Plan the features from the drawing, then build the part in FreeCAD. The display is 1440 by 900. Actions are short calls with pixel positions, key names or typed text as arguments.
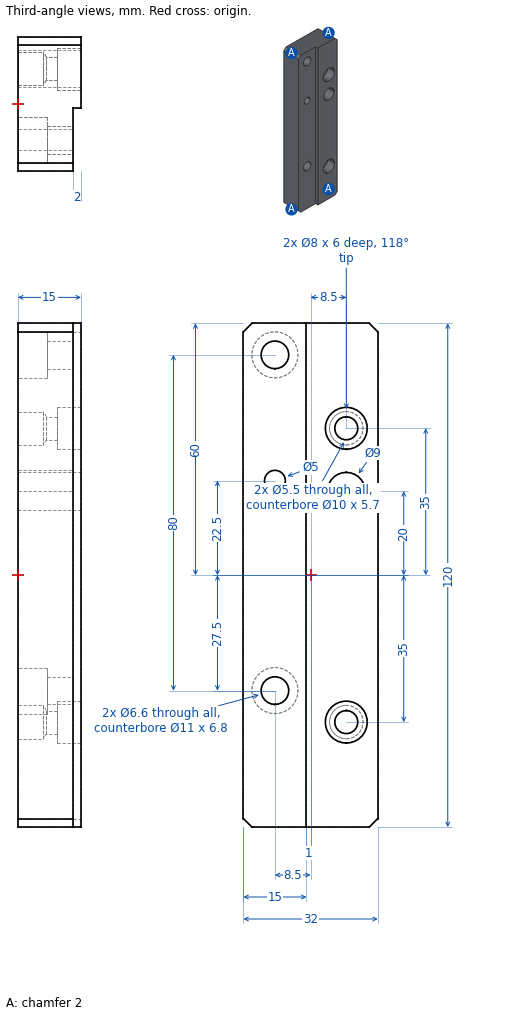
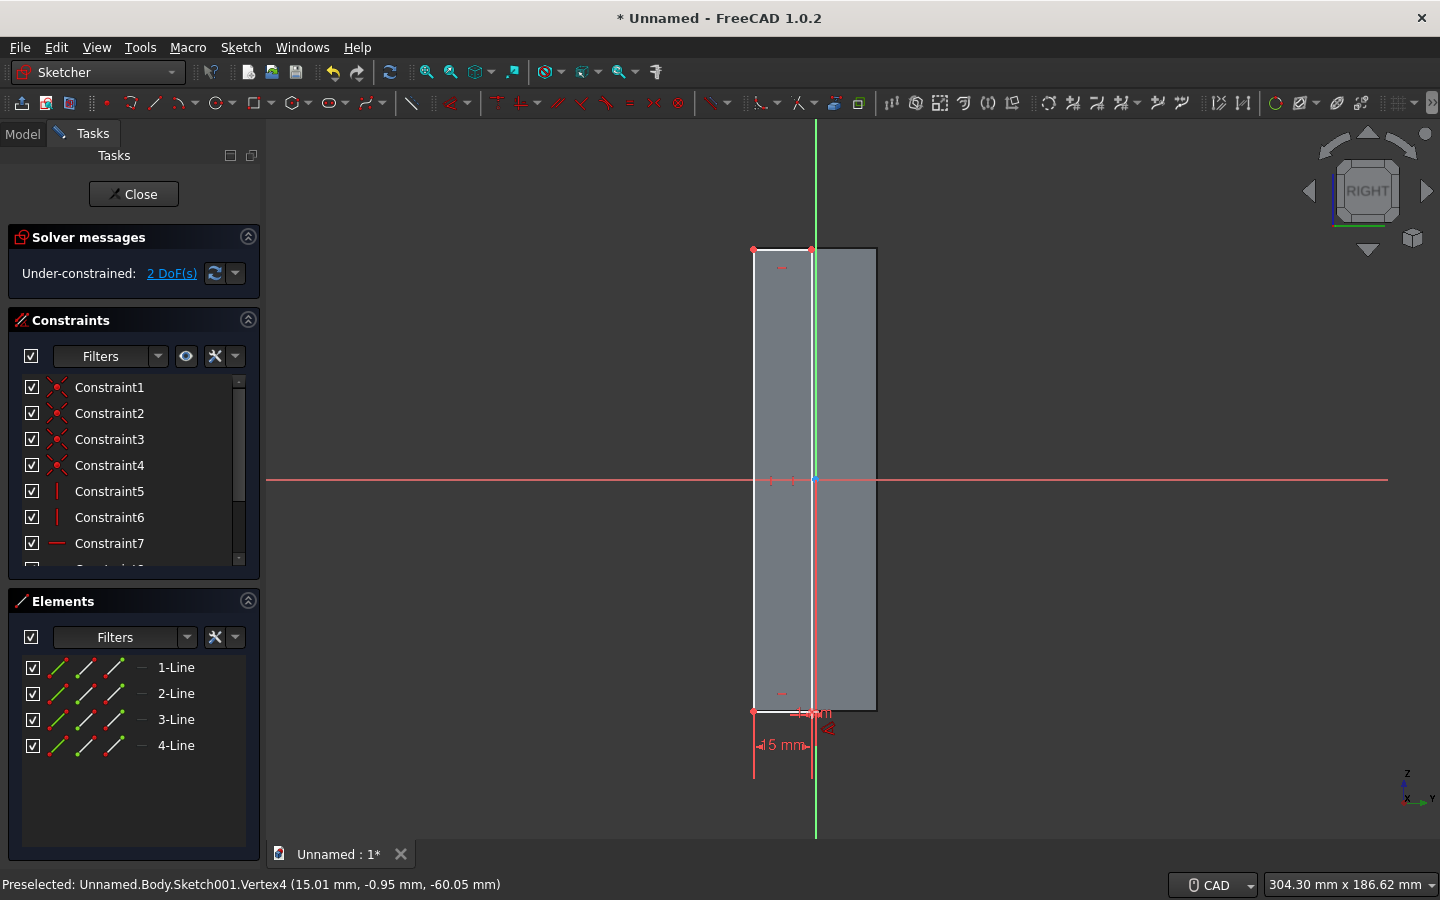
click(754, 388)
click(720, 374)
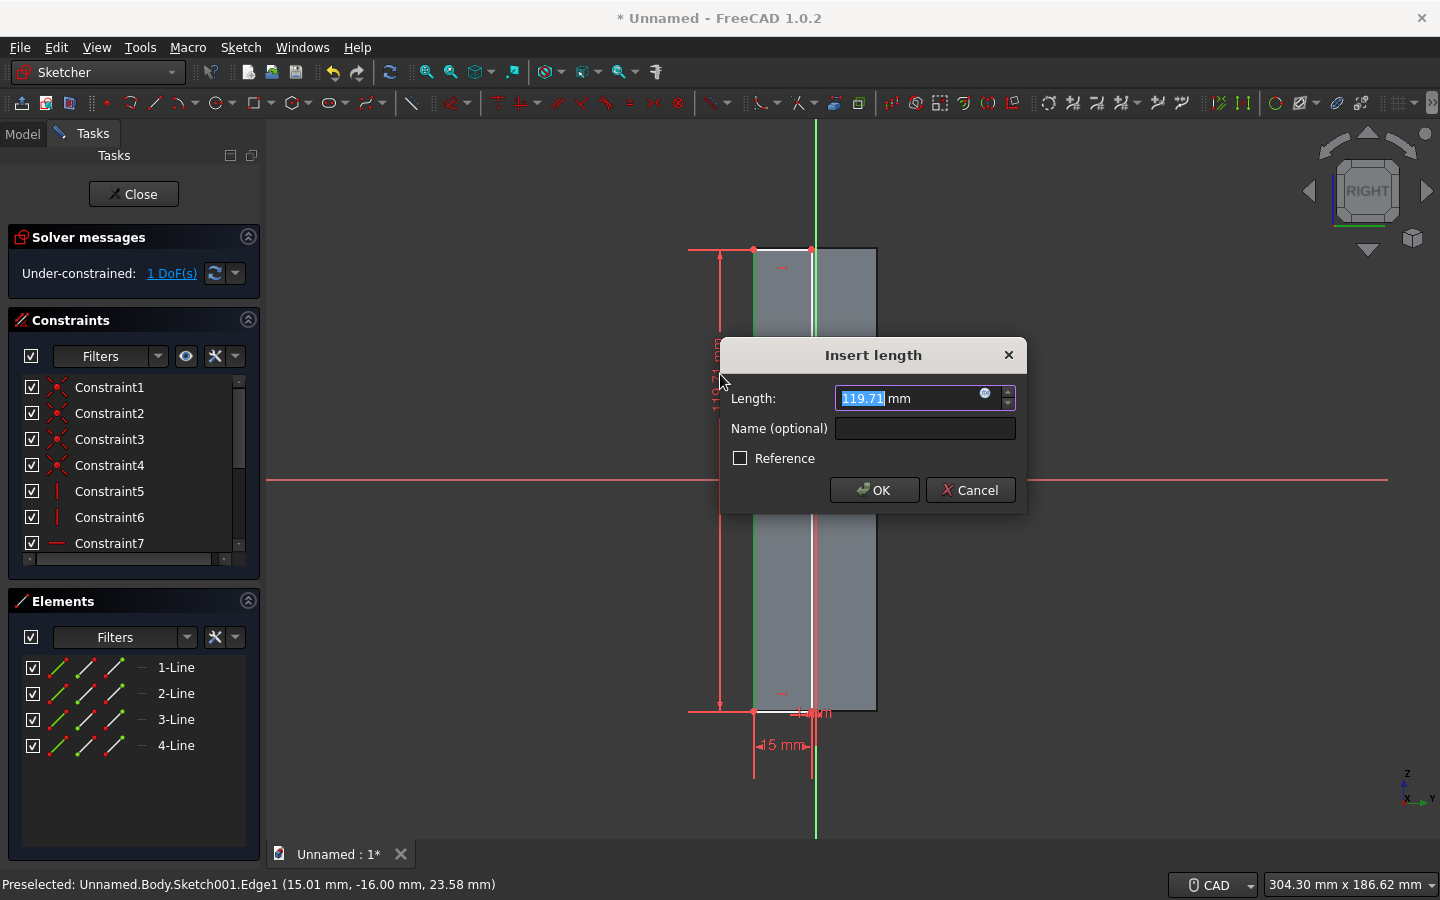
text(120)
key(Return)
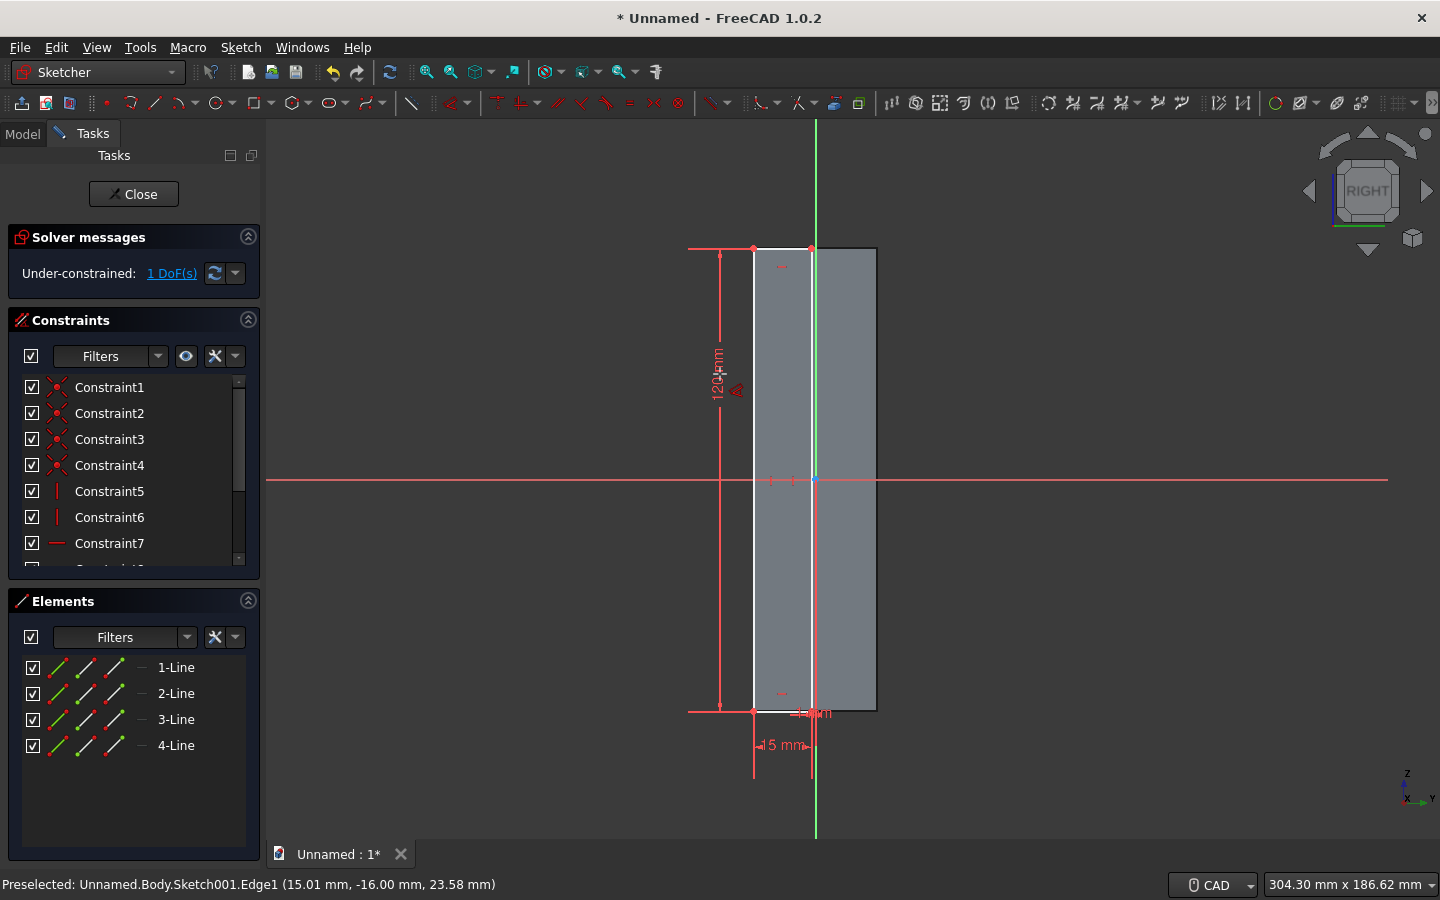
click(754, 249)
click(850, 364)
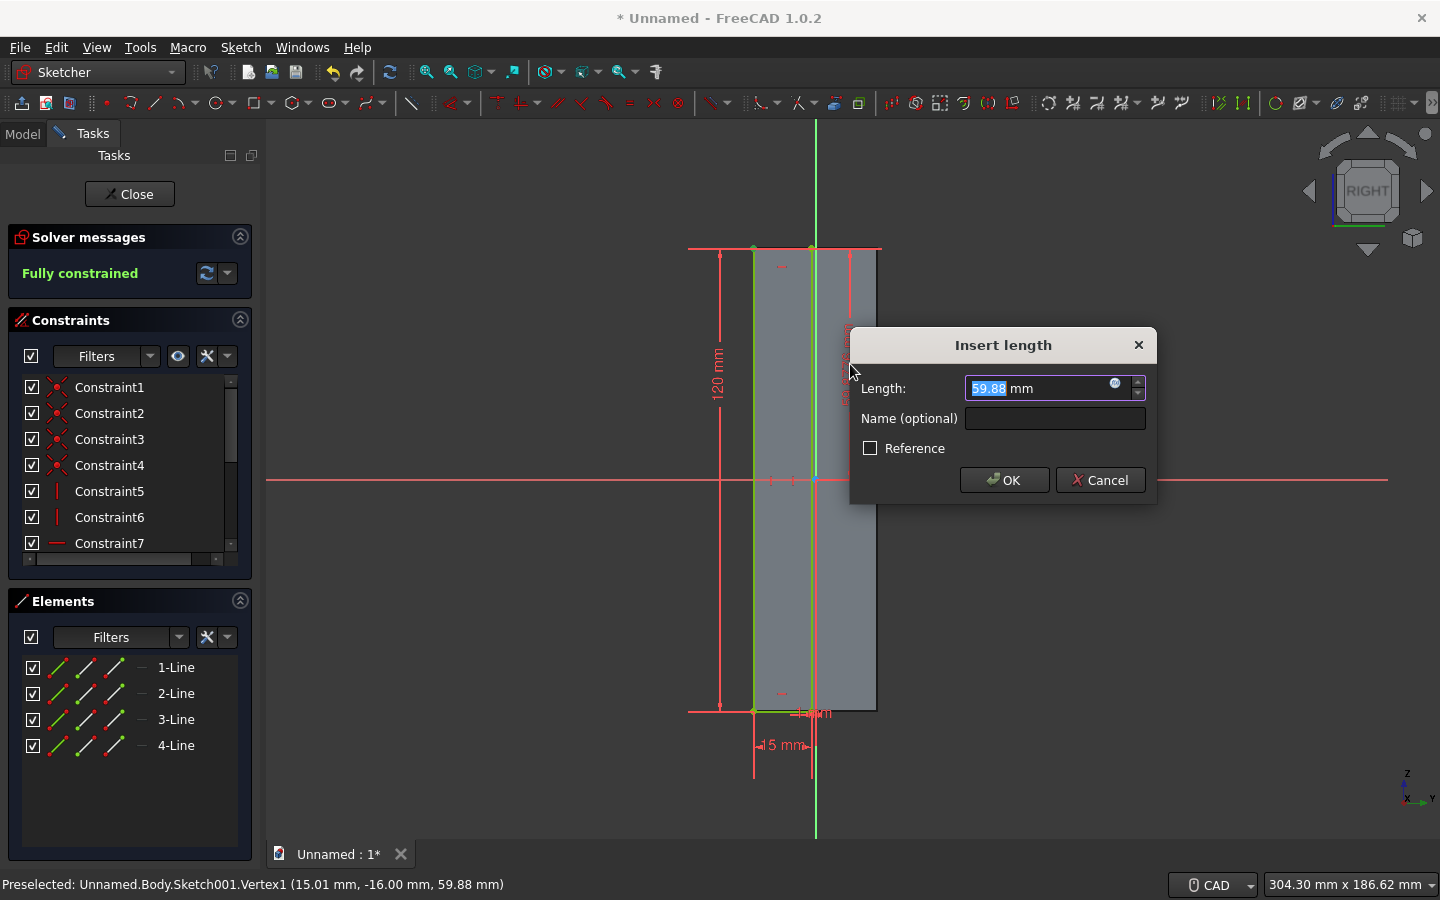
text(60)
key(Return)
key(Escape)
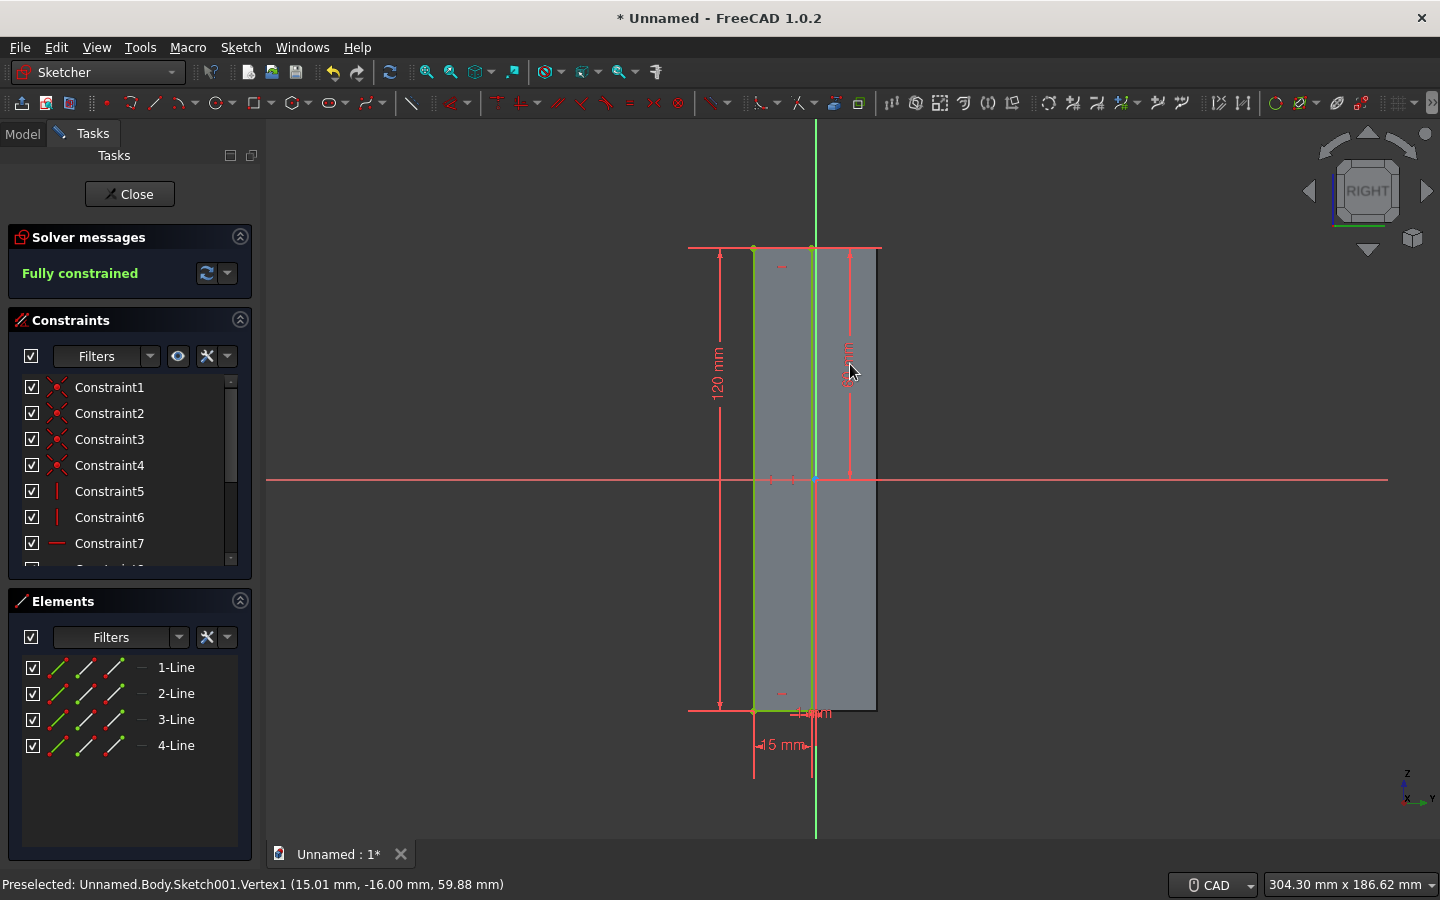
click(130, 194)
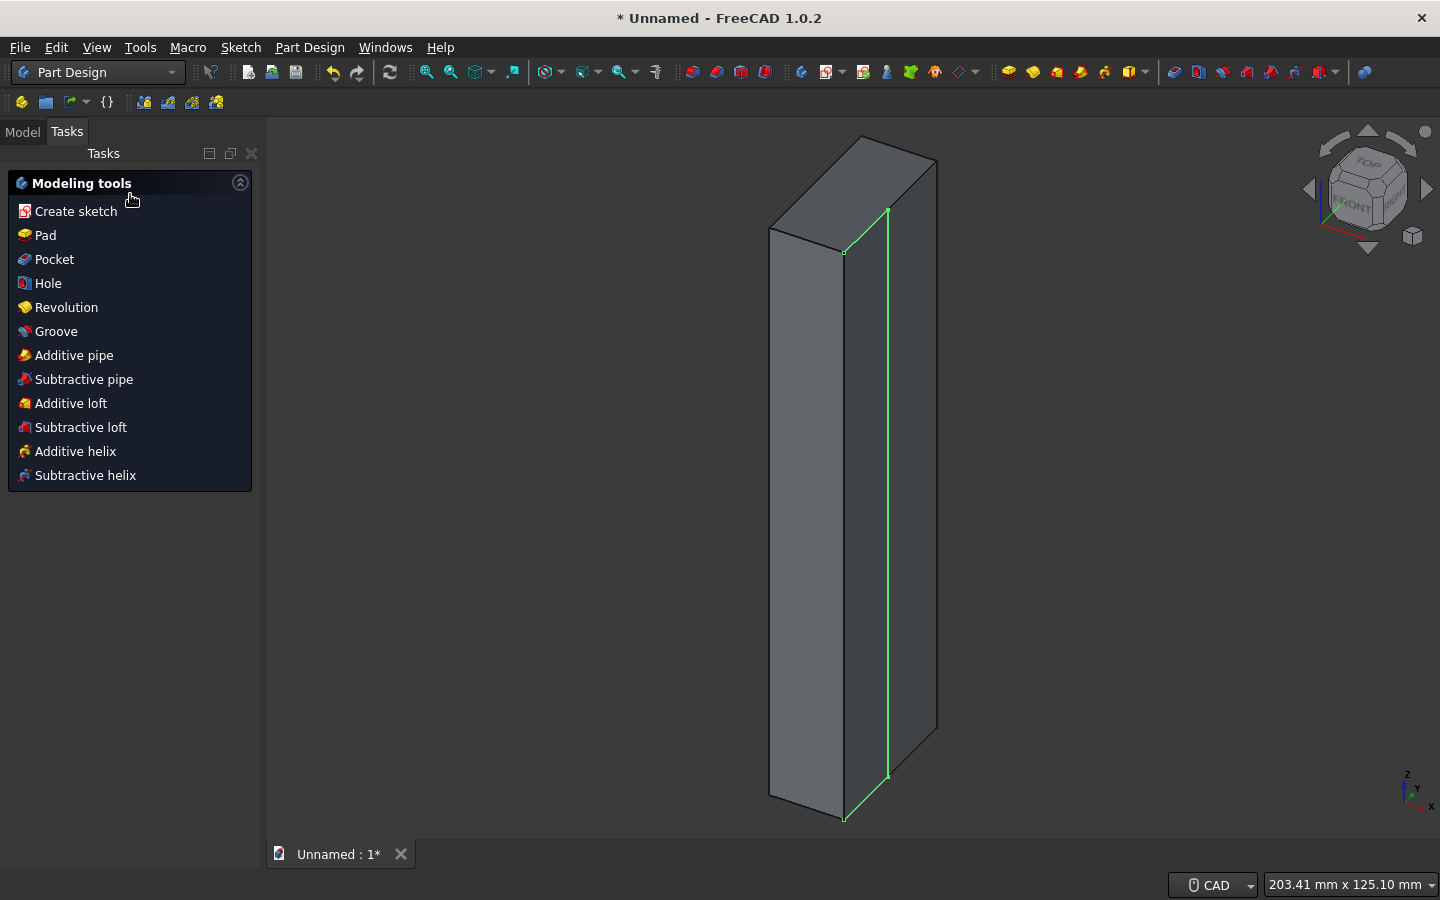
click(1176, 72)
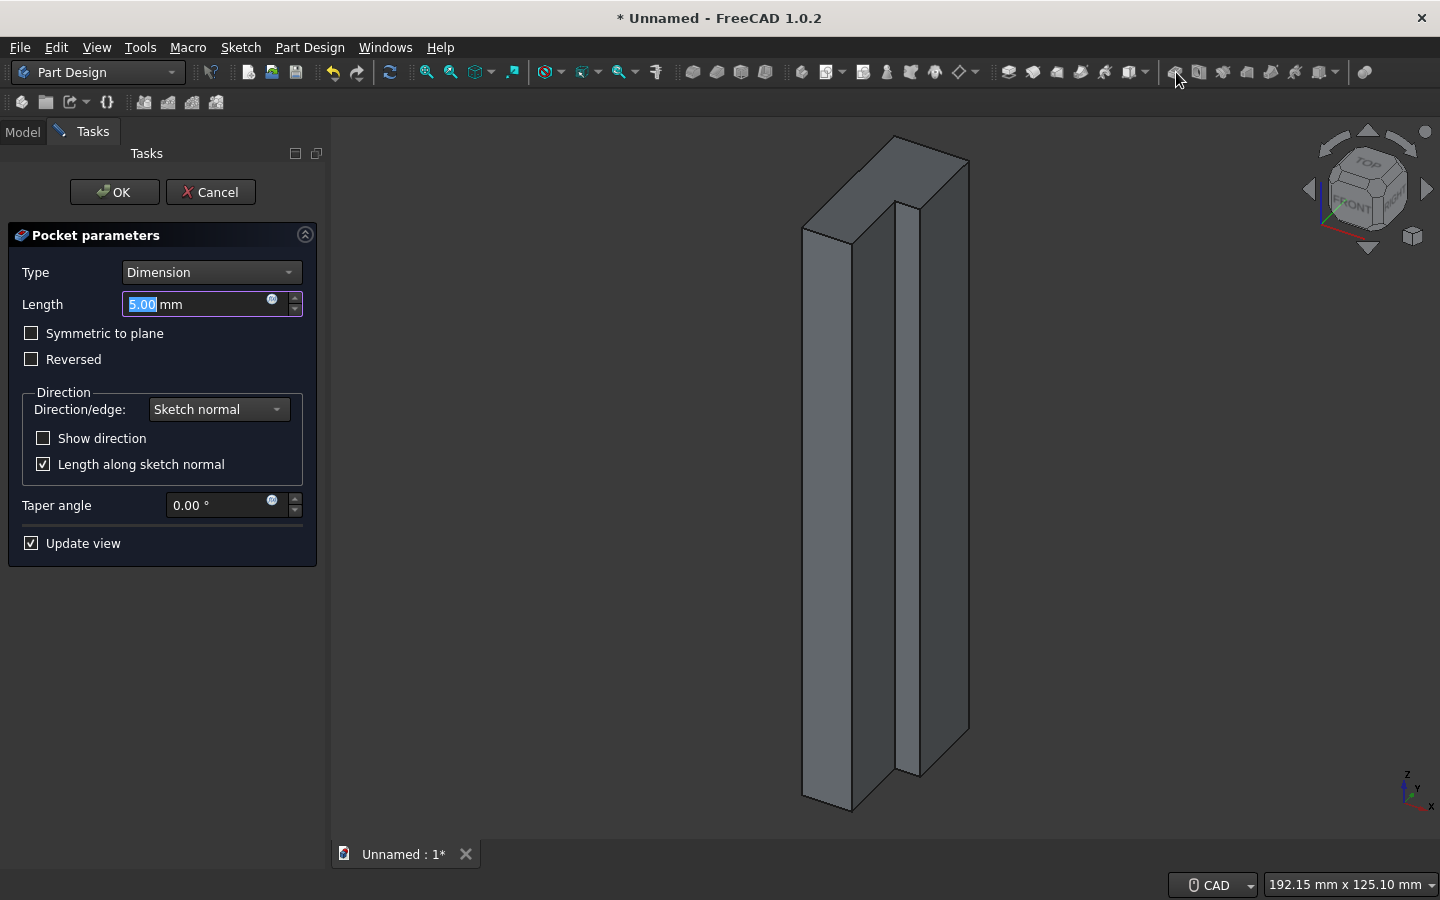
text(2)
key(Tab)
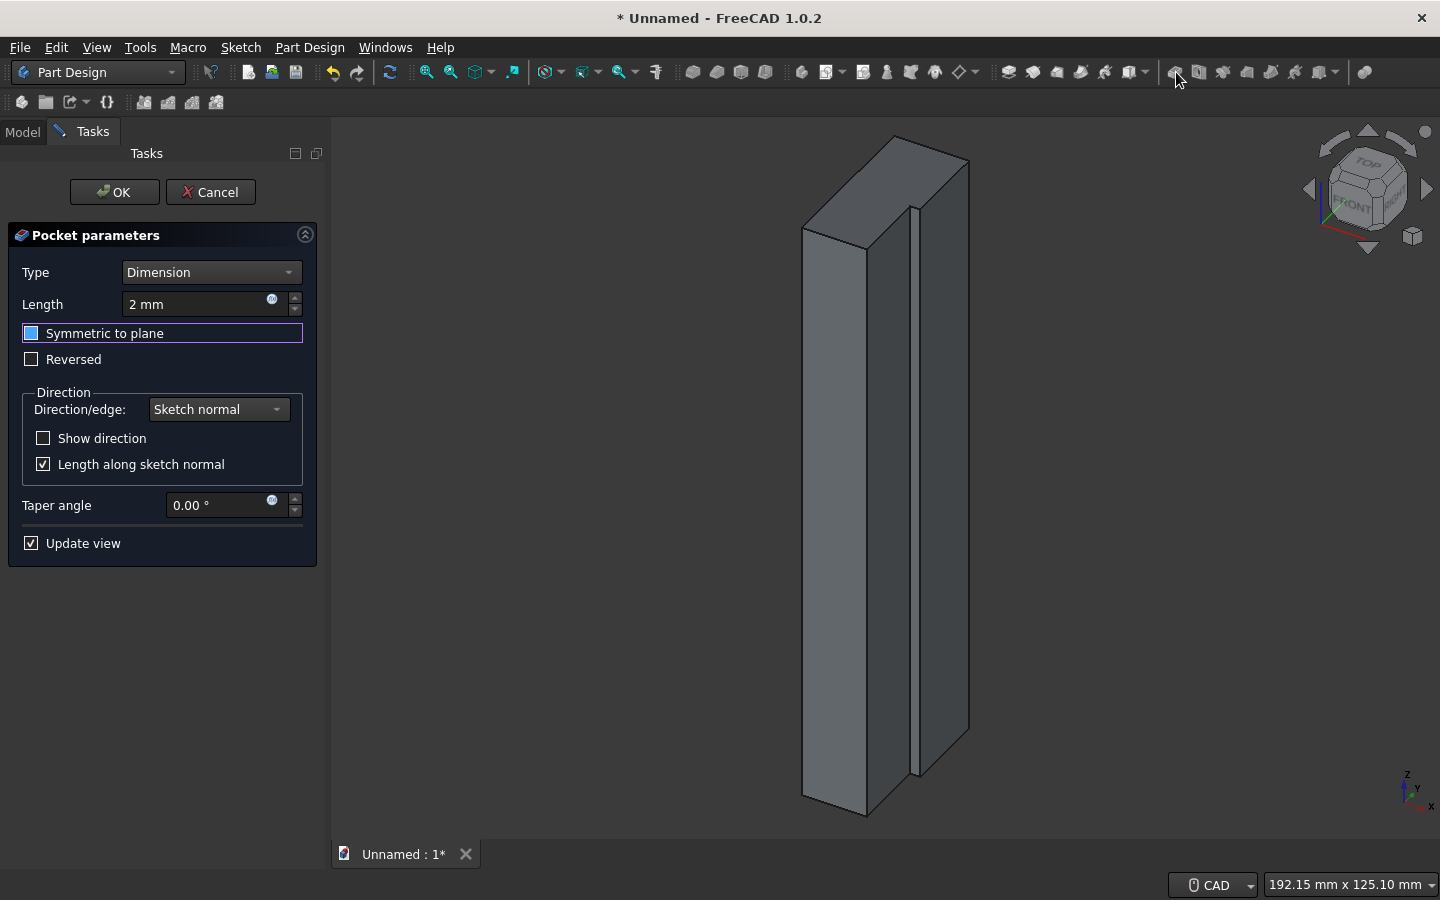
click(115, 192)